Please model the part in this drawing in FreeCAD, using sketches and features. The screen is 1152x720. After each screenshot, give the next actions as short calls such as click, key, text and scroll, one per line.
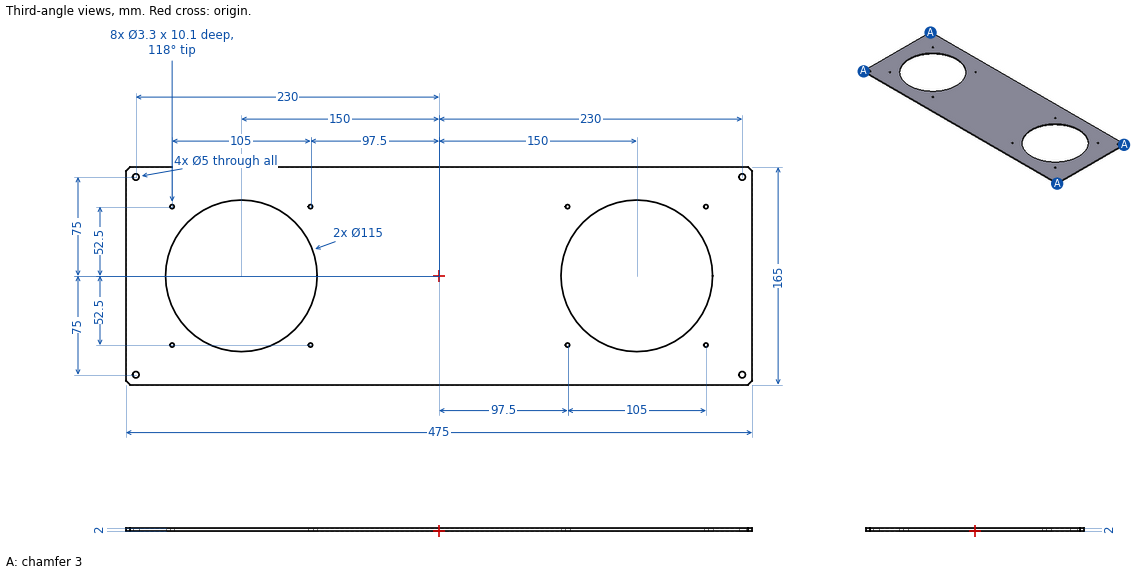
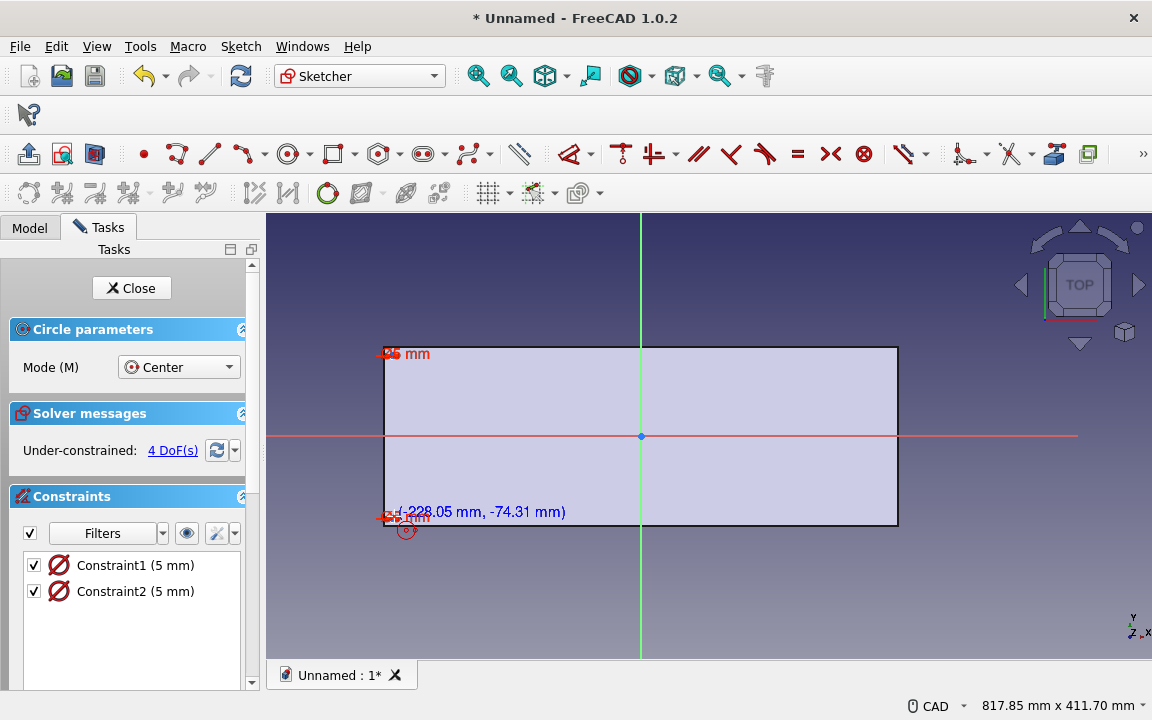
scroll(890, 355, up, 11)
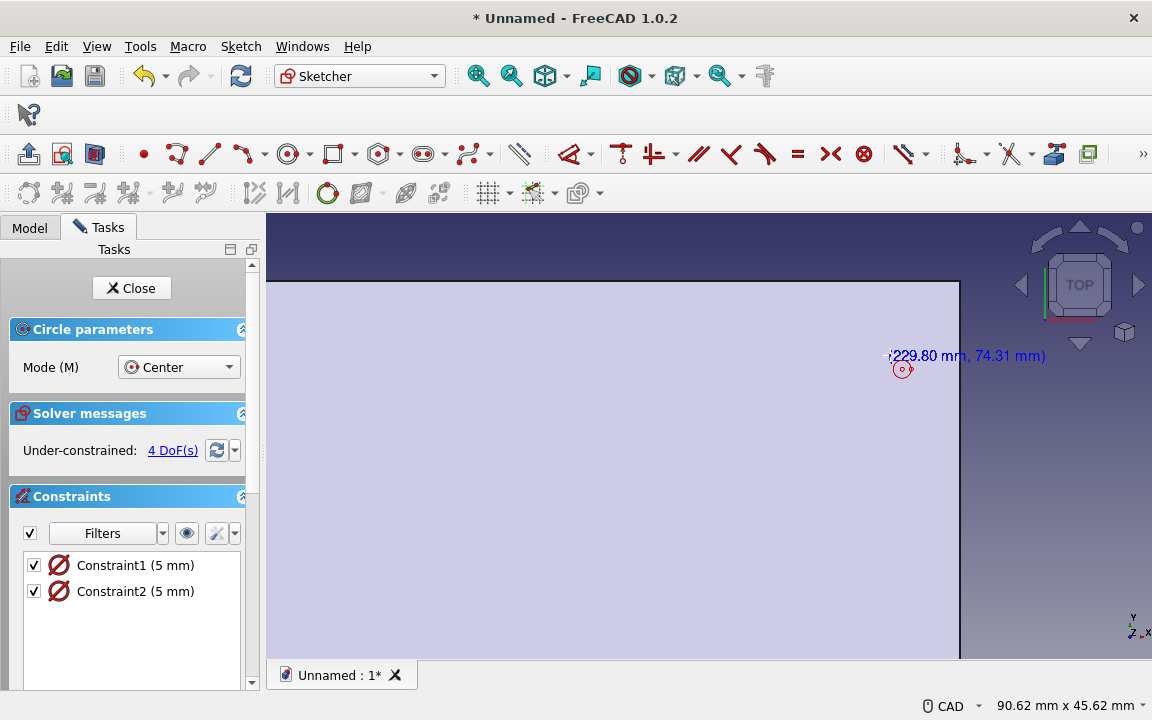
scroll(890, 355, down, 11)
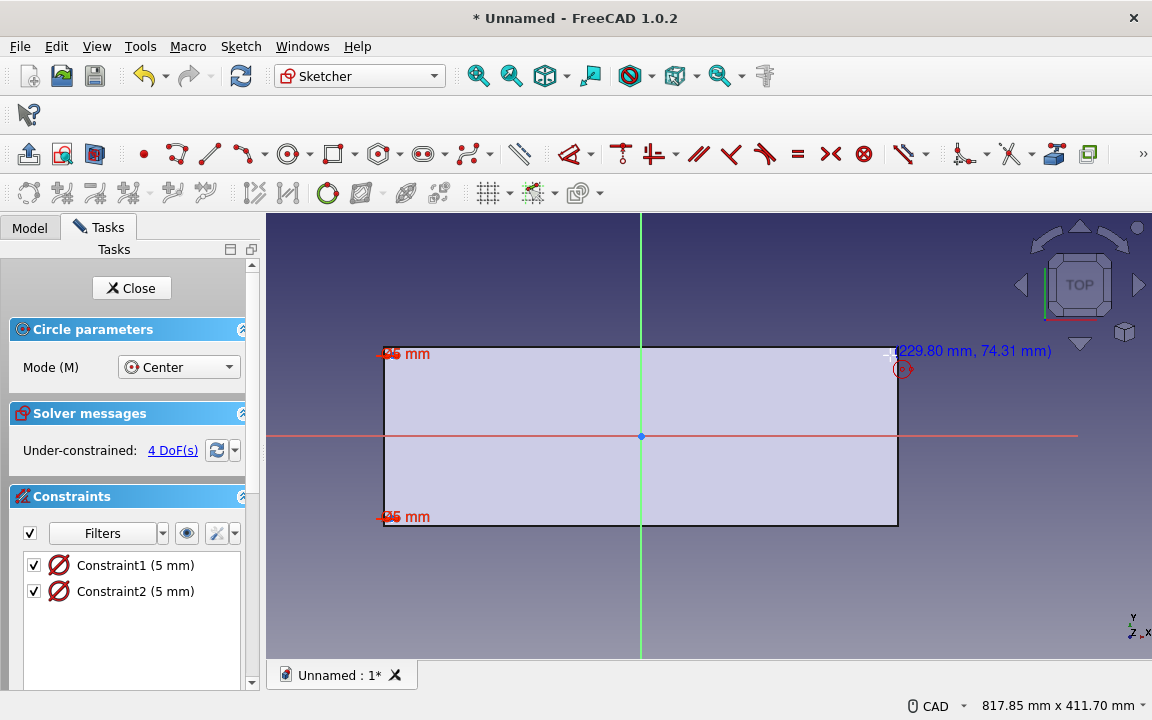
click(890, 355)
move(892, 353)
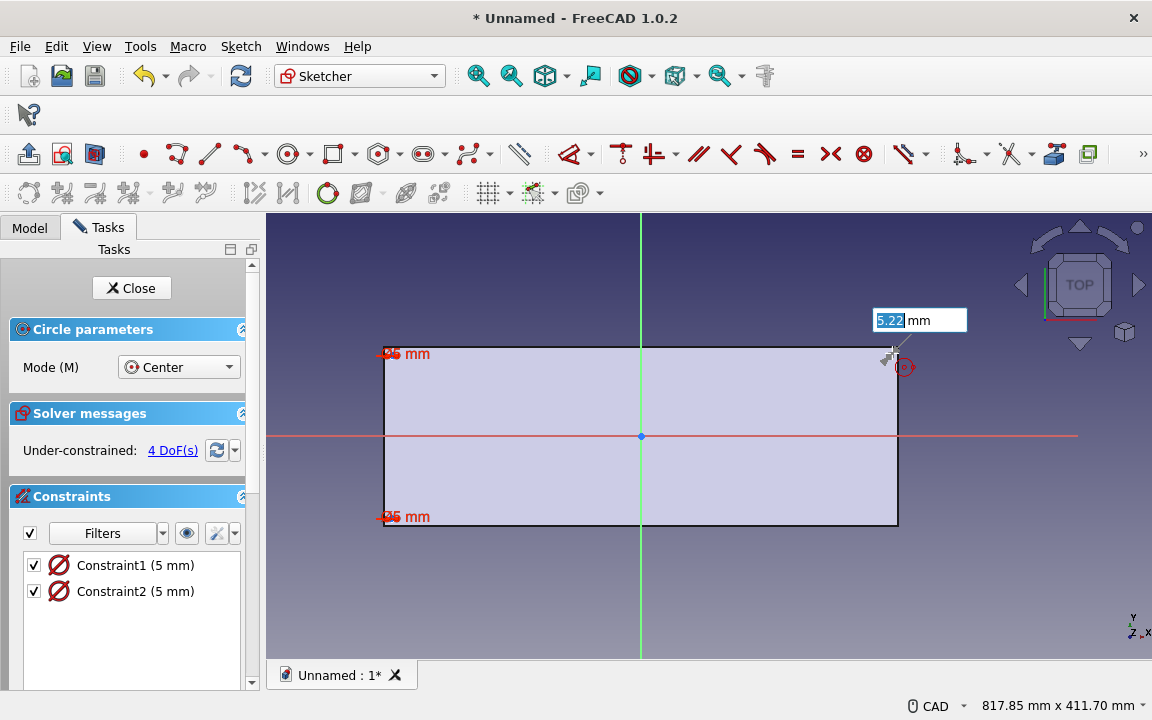
text(5)
key(Return)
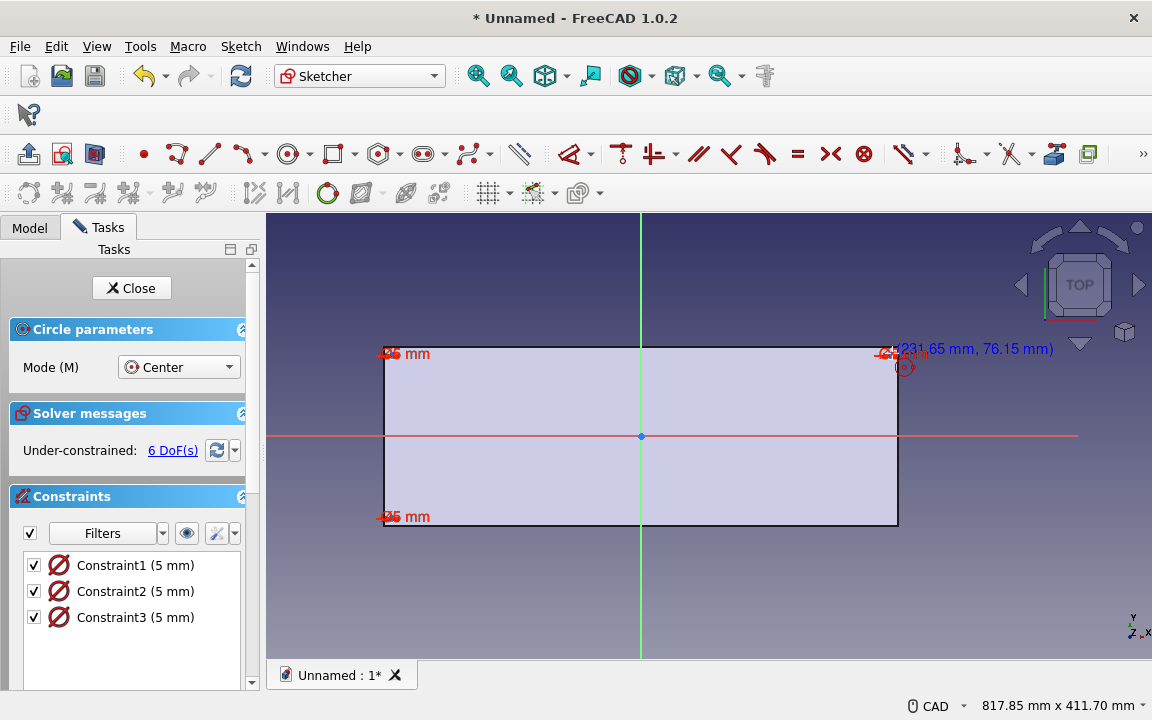
scroll(890, 518, up, 11)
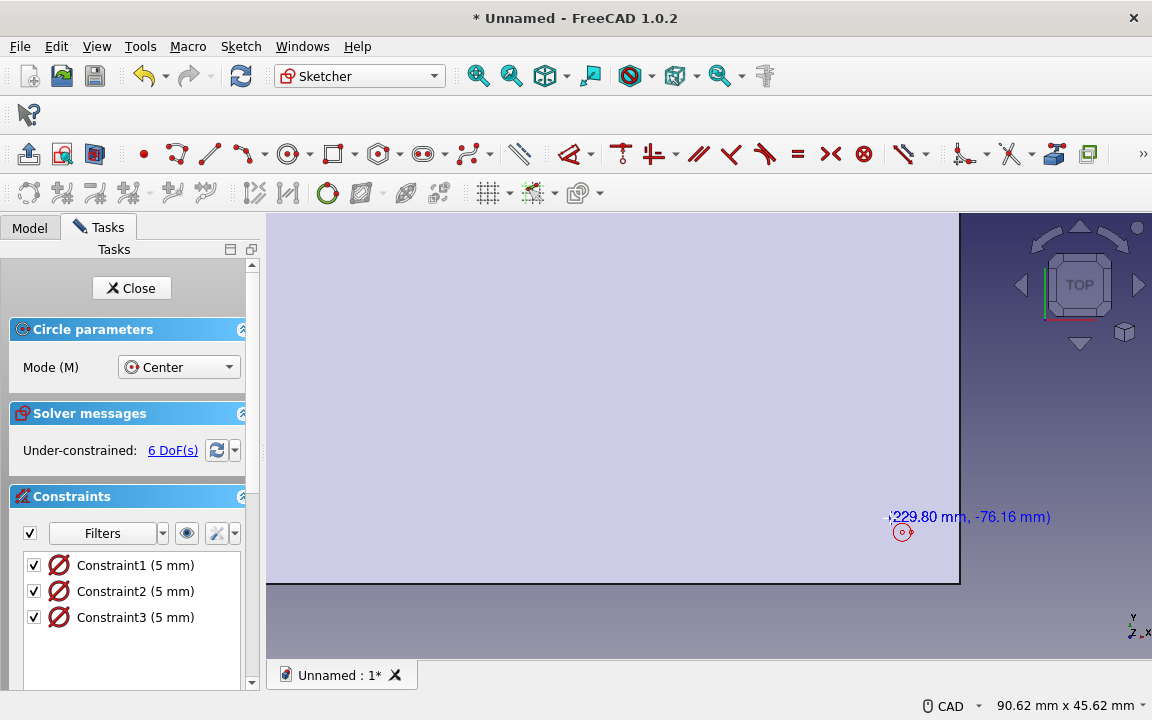
scroll(890, 518, down, 11)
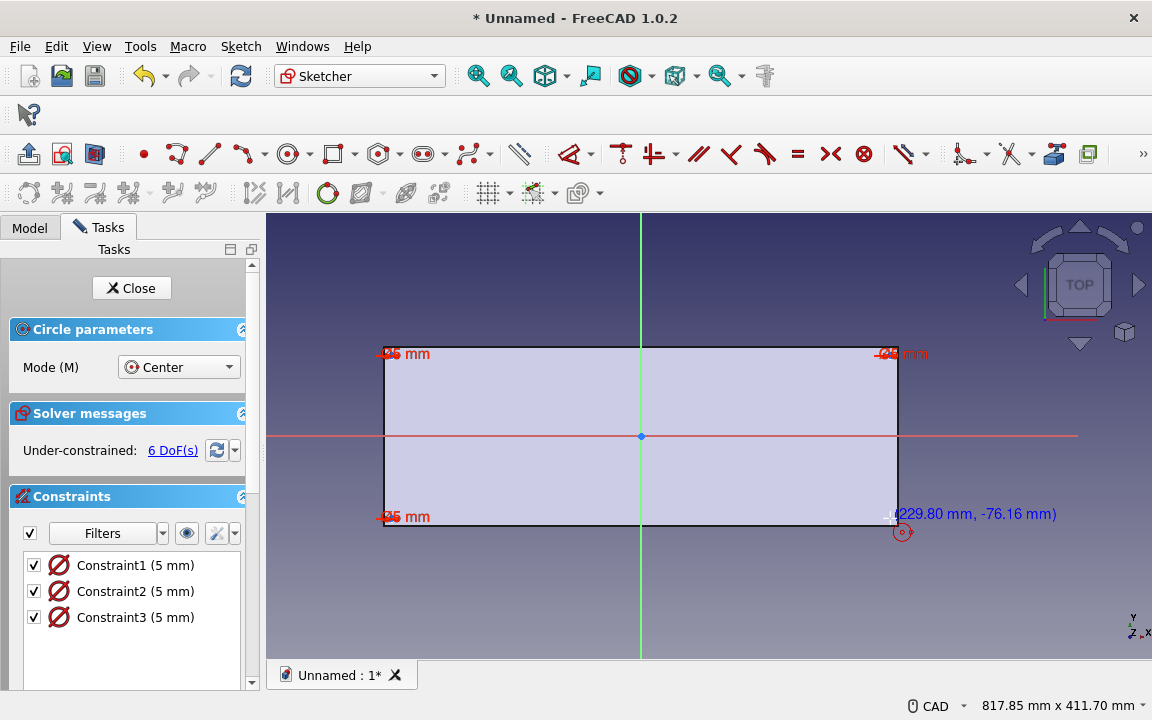
click(890, 518)
move(892, 516)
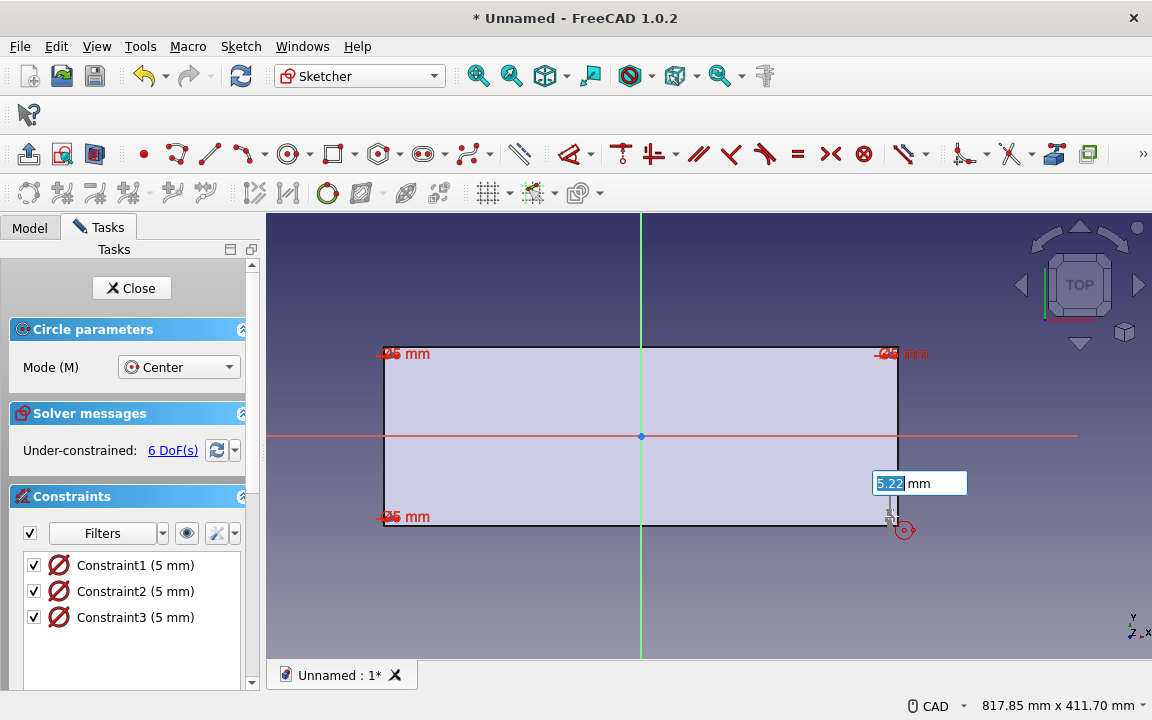
text(5)
key(Return)
key(Escape)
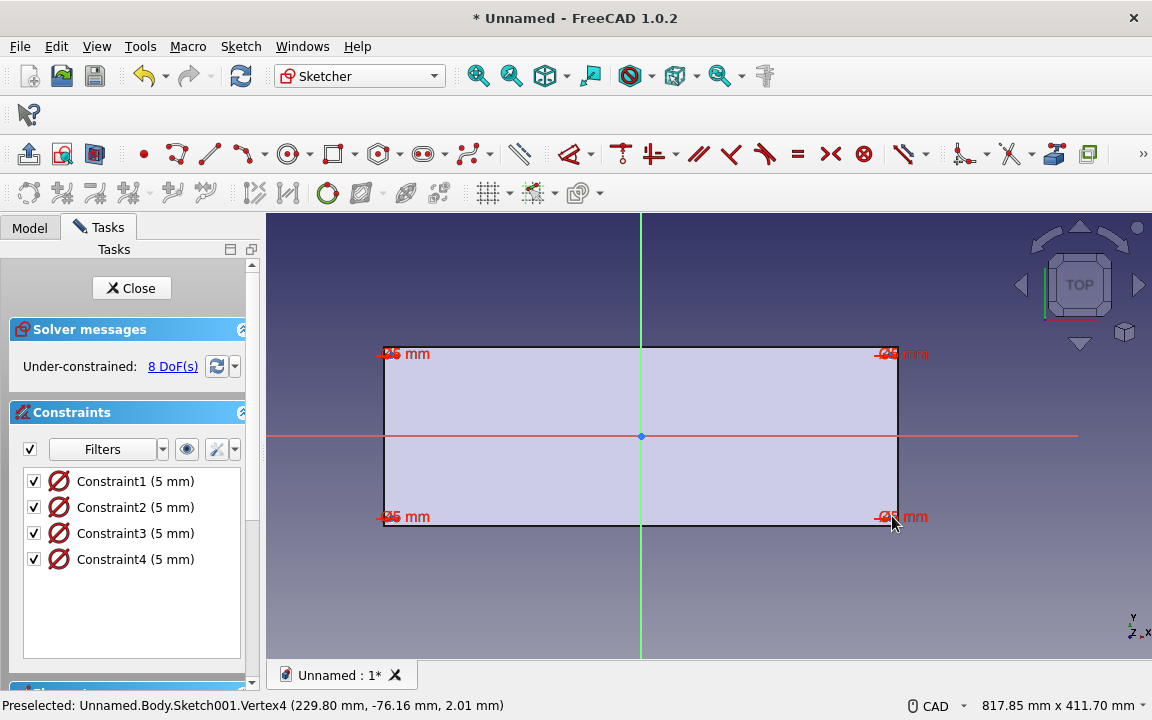
click(392, 356)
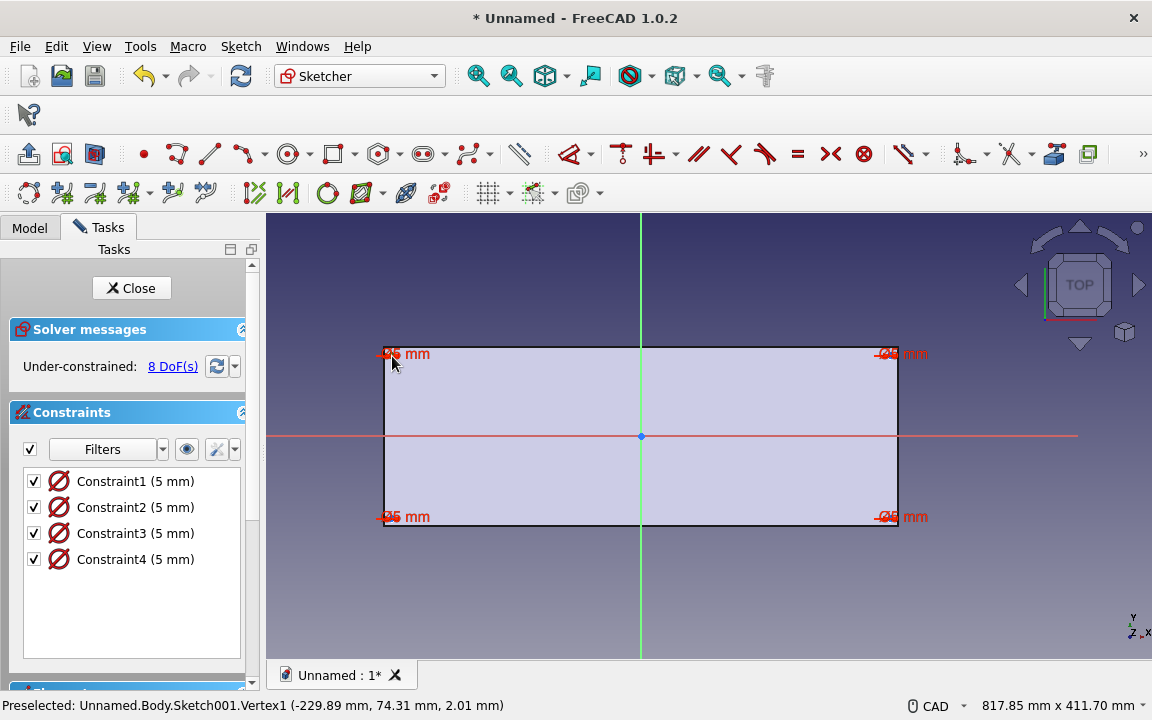
click(392, 519)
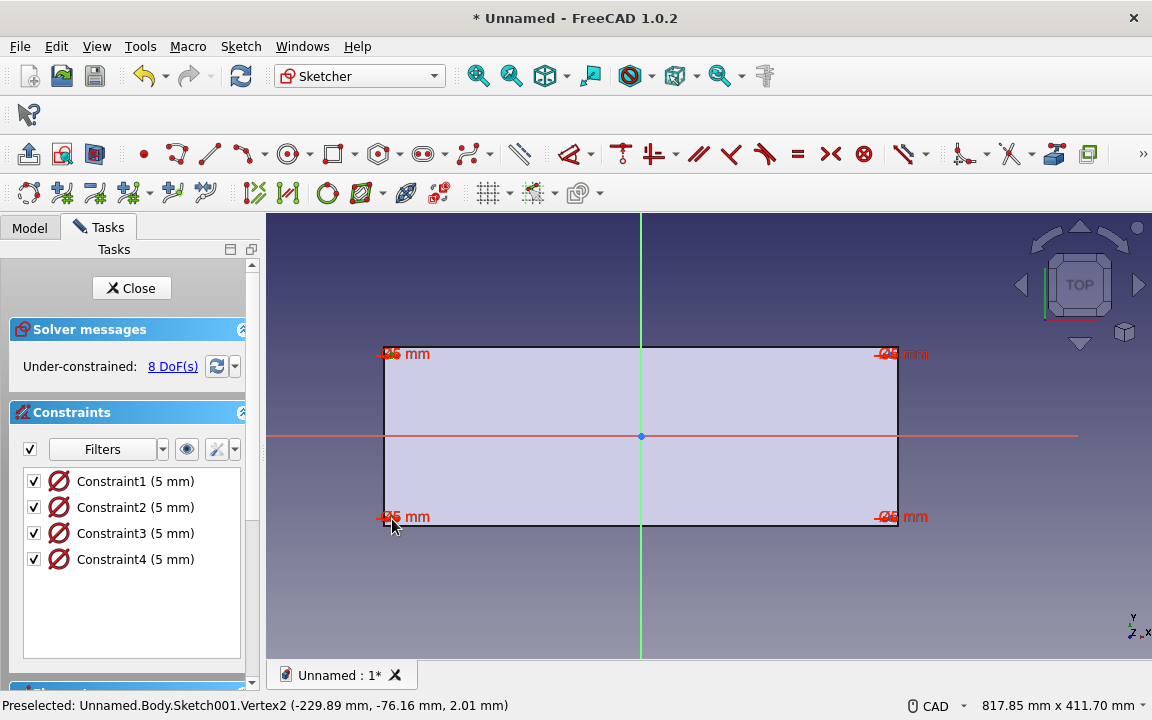
key(v)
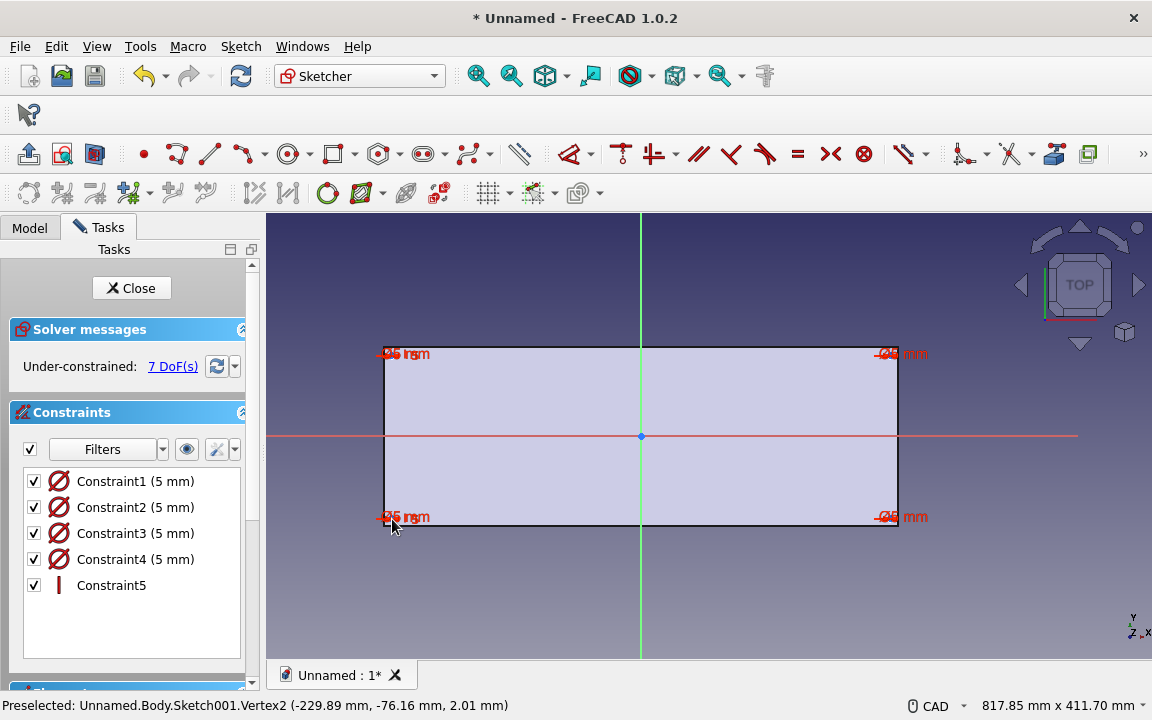
click(392, 356)